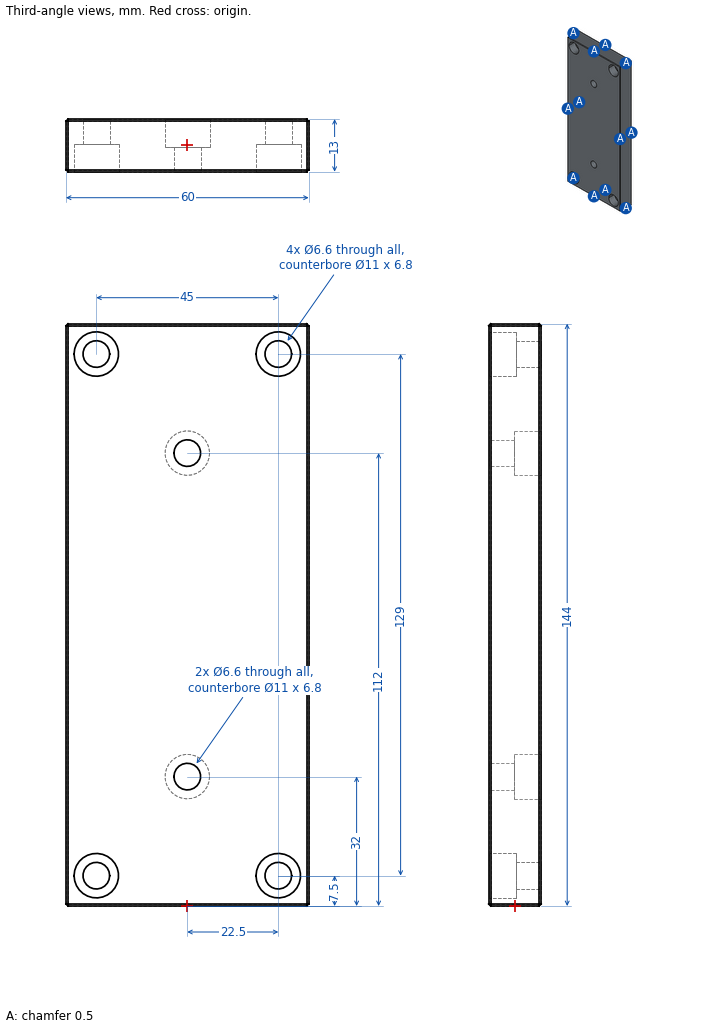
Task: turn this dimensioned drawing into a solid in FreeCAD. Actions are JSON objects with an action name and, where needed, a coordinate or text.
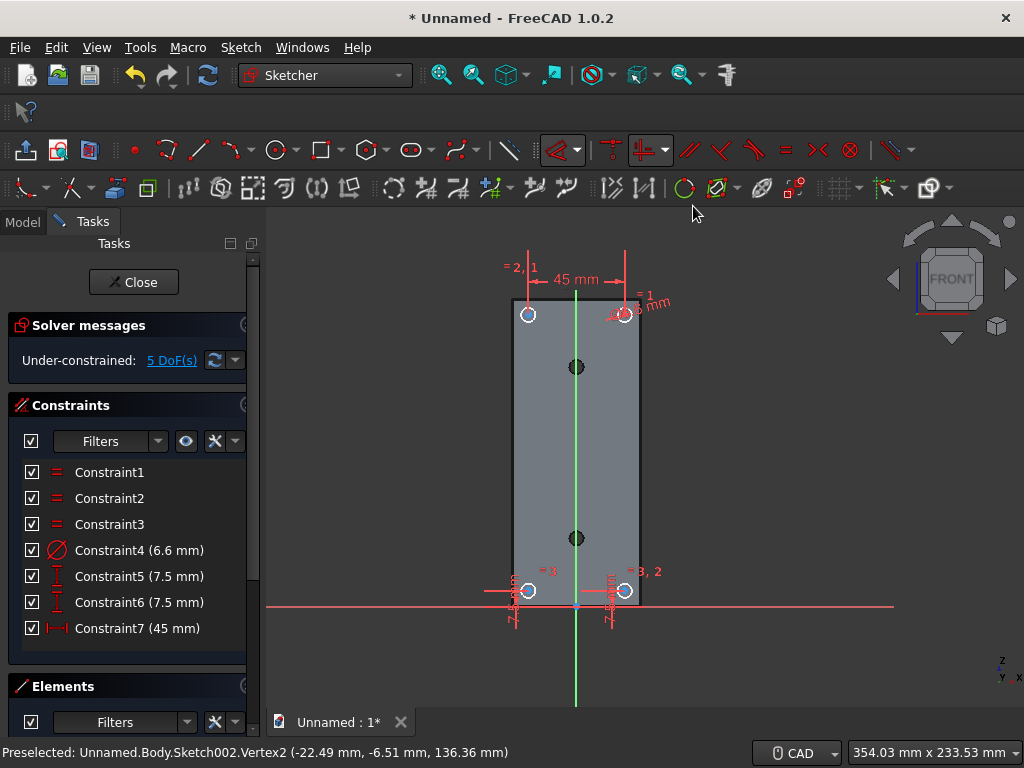
{"action": "left_click", "coordinate": [528, 315]}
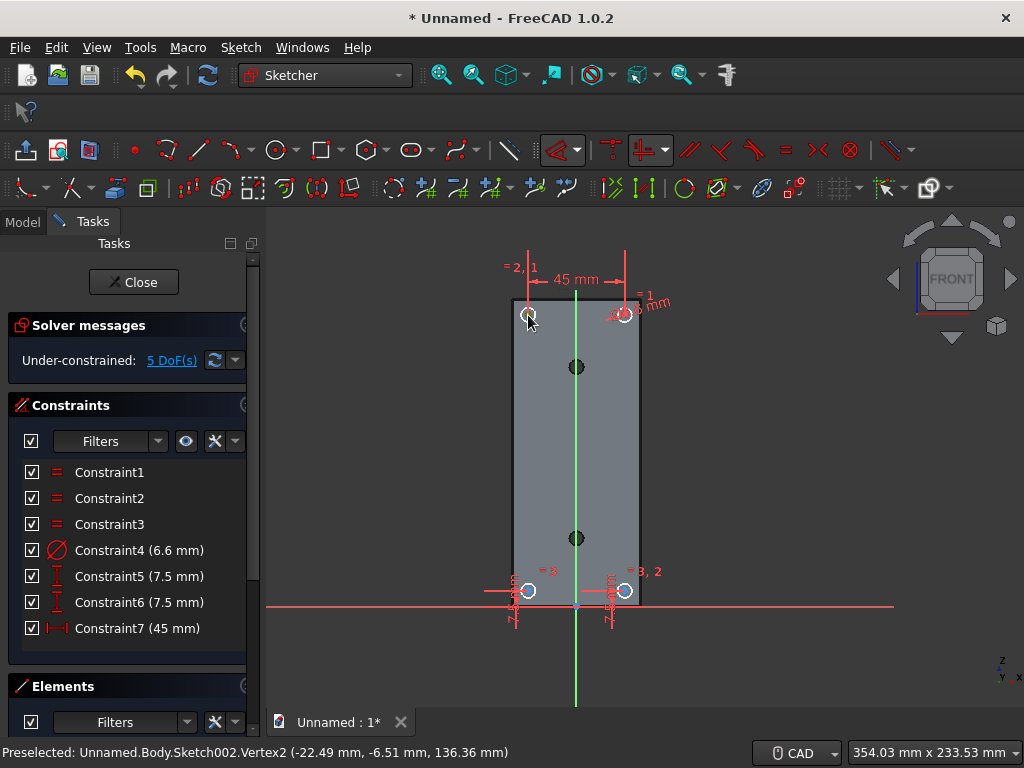
{"action": "left_click", "coordinate": [625, 591]}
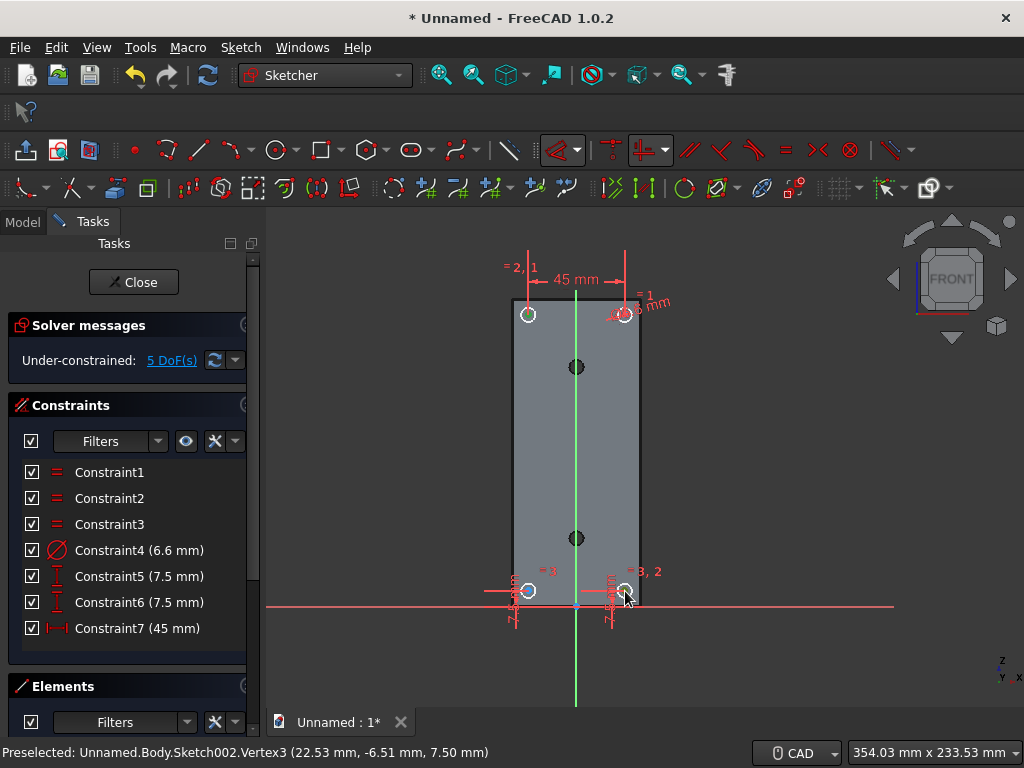
{"action": "left_click", "coordinate": [580, 150]}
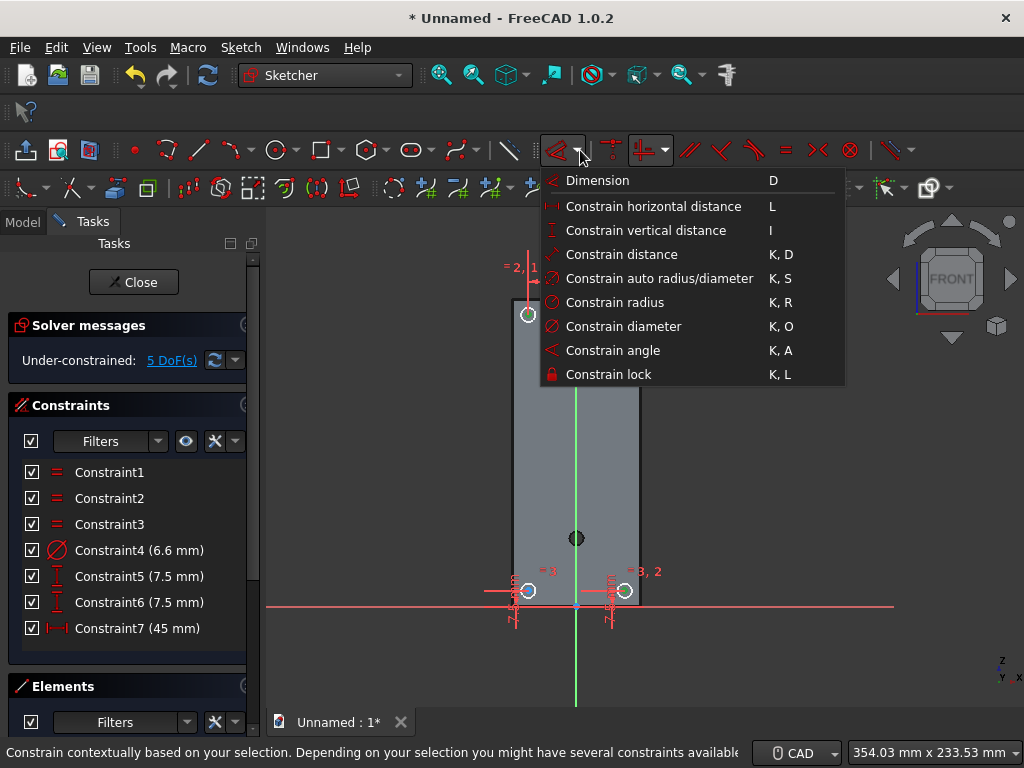
{"action": "left_click", "coordinate": [693, 206]}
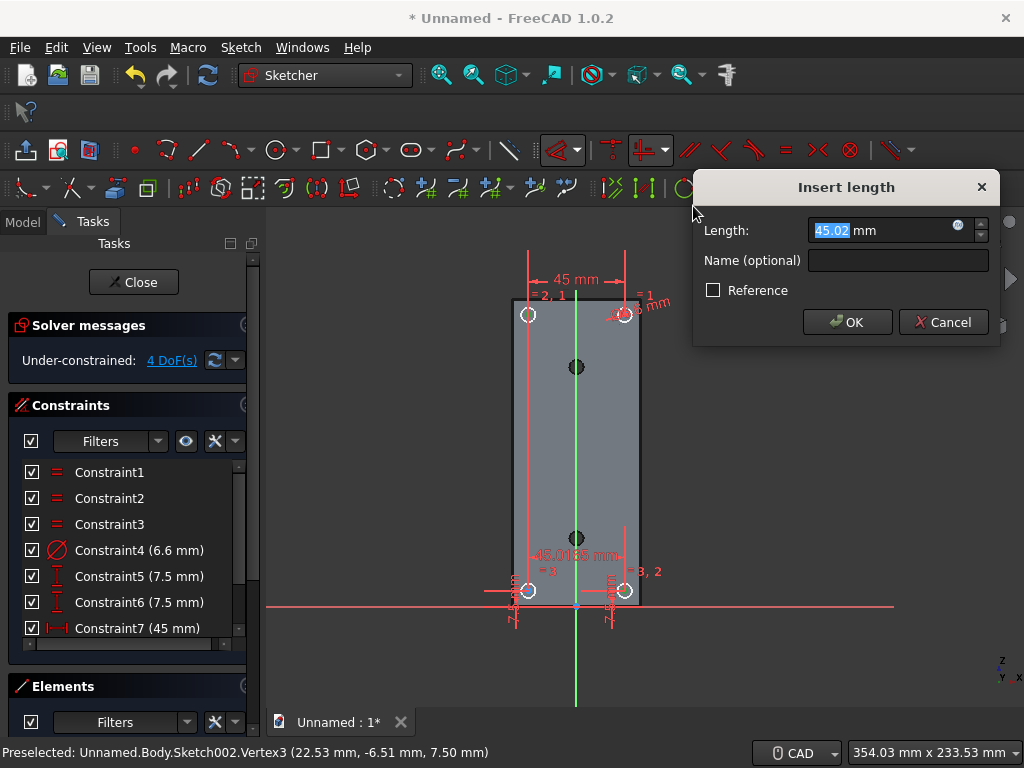
{"action": "type", "text": "45"}
{"action": "key", "text": "Return"}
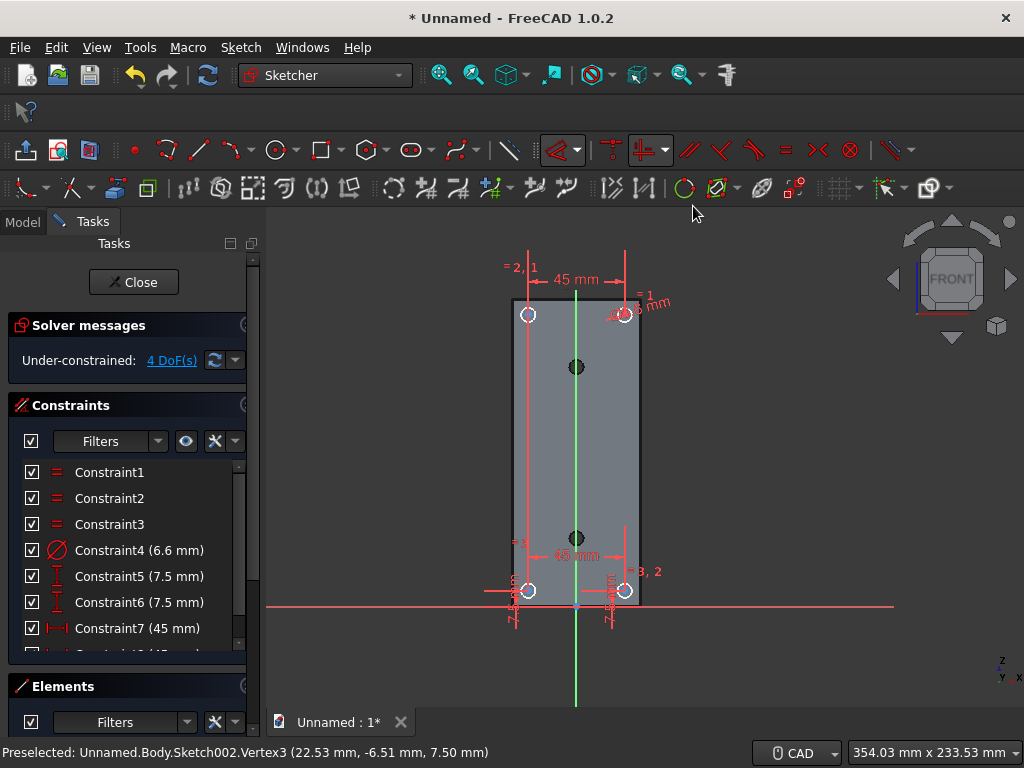
{"action": "left_click", "coordinate": [625, 591]}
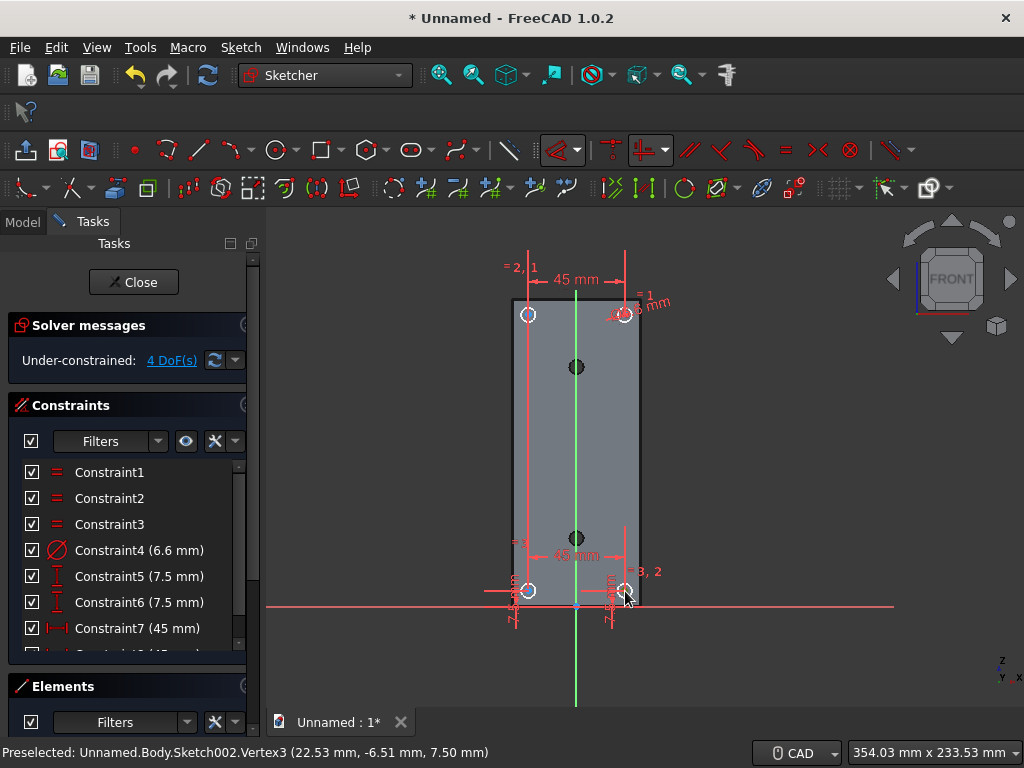
{"action": "left_click", "coordinate": [528, 591]}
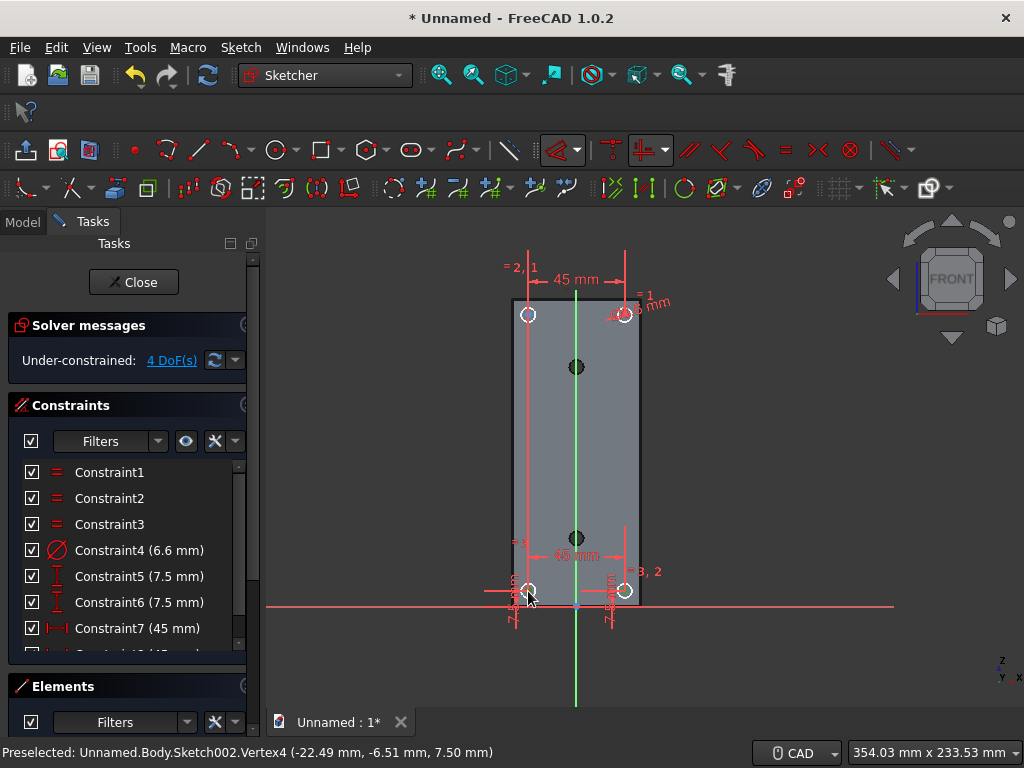
{"action": "key", "text": "l"}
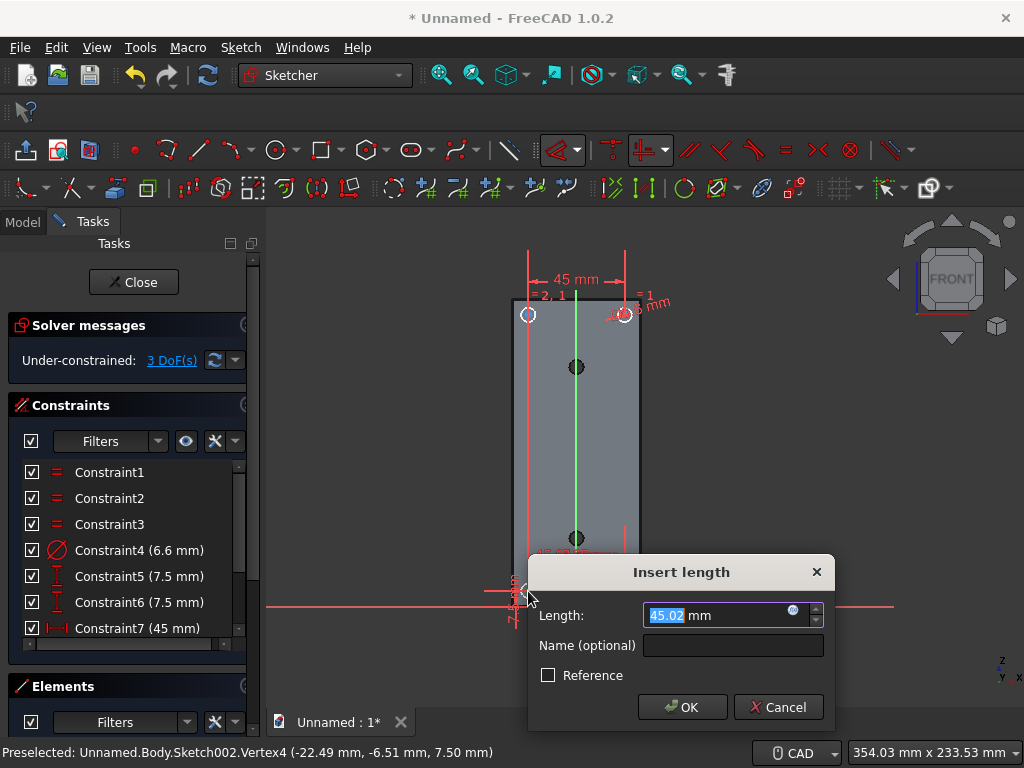
{"action": "type", "text": "45"}
{"action": "key", "text": "Return"}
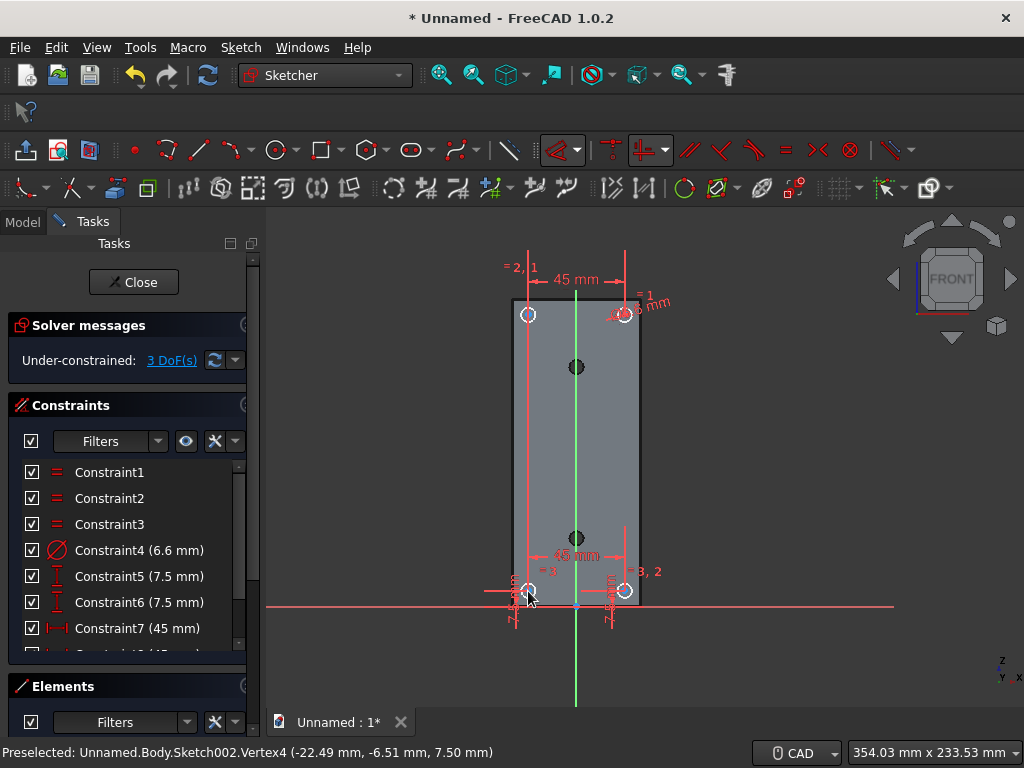
{"action": "left_click", "coordinate": [625, 315]}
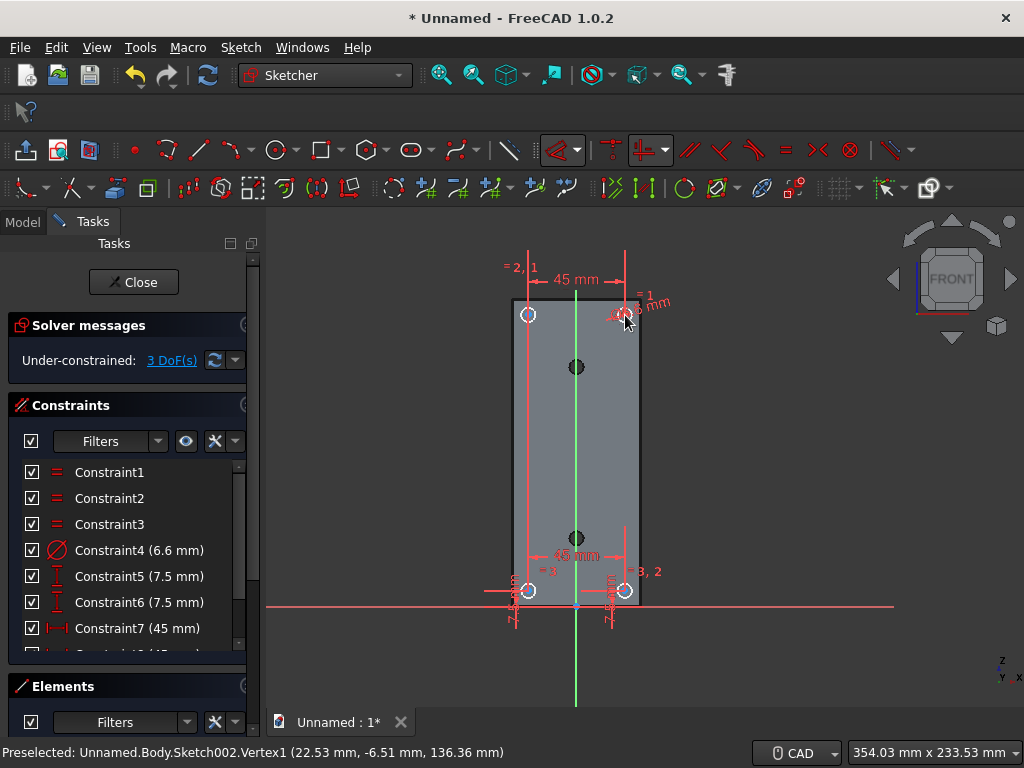
{"action": "key", "text": "l"}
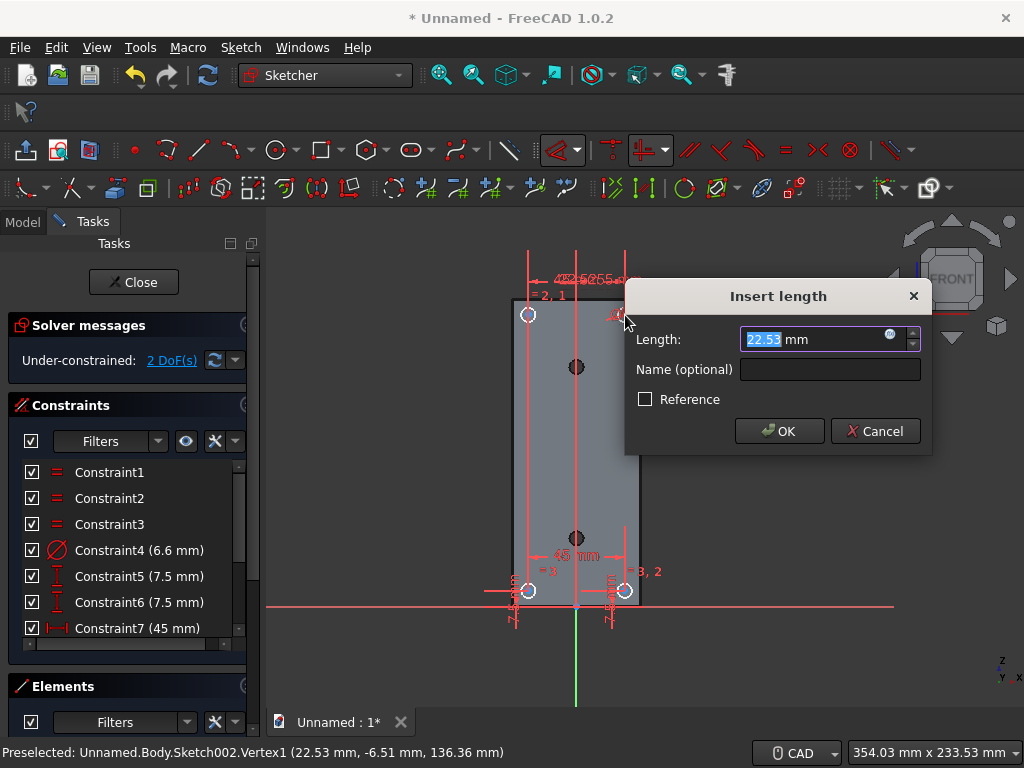
{"action": "type", "text": "22.5"}
{"action": "key", "text": "Return"}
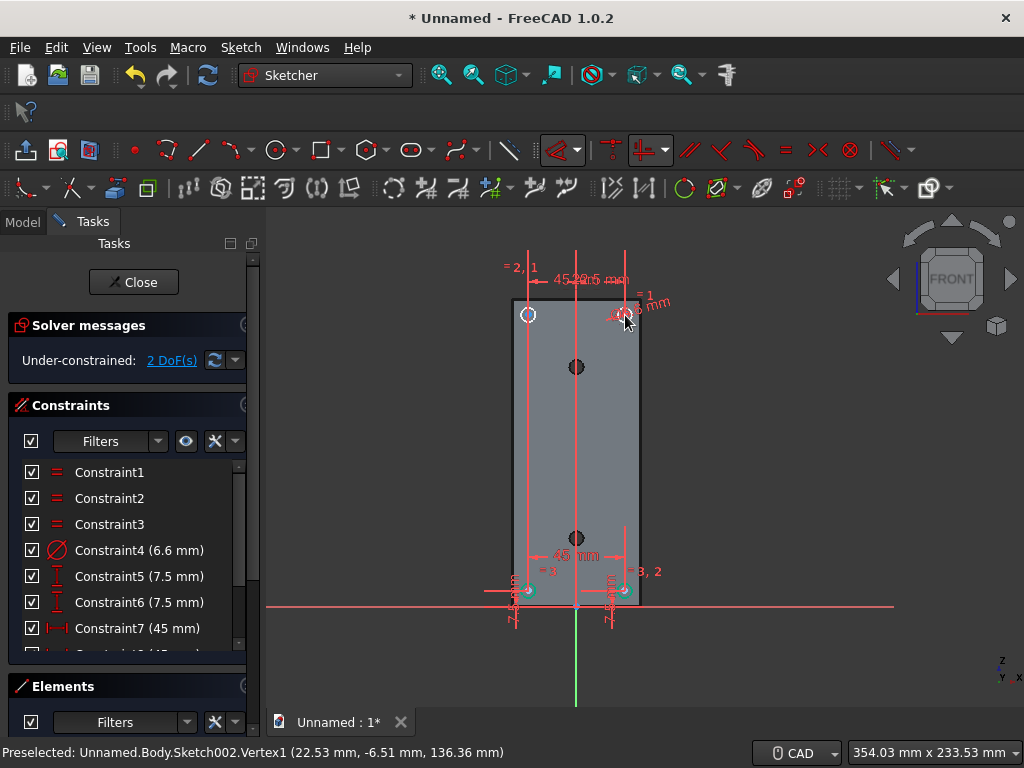
{"action": "left_click", "coordinate": [625, 315]}